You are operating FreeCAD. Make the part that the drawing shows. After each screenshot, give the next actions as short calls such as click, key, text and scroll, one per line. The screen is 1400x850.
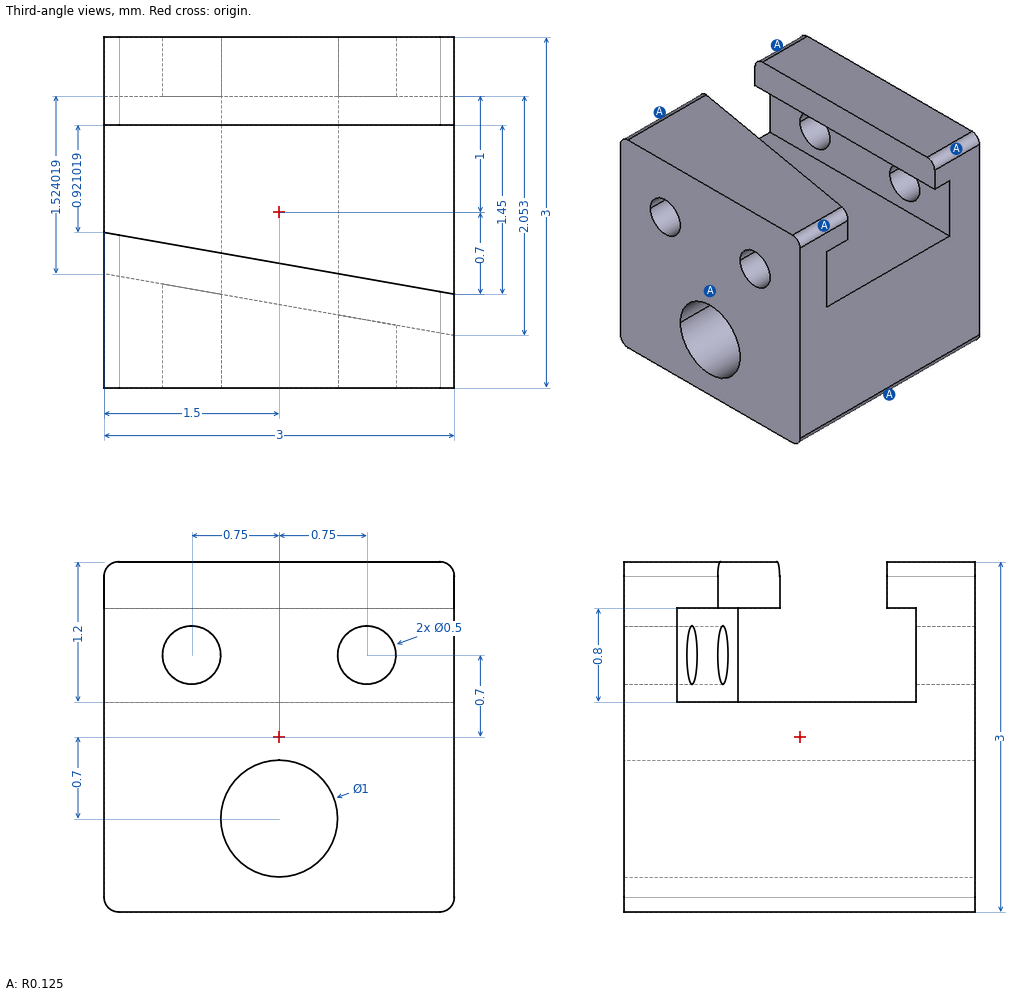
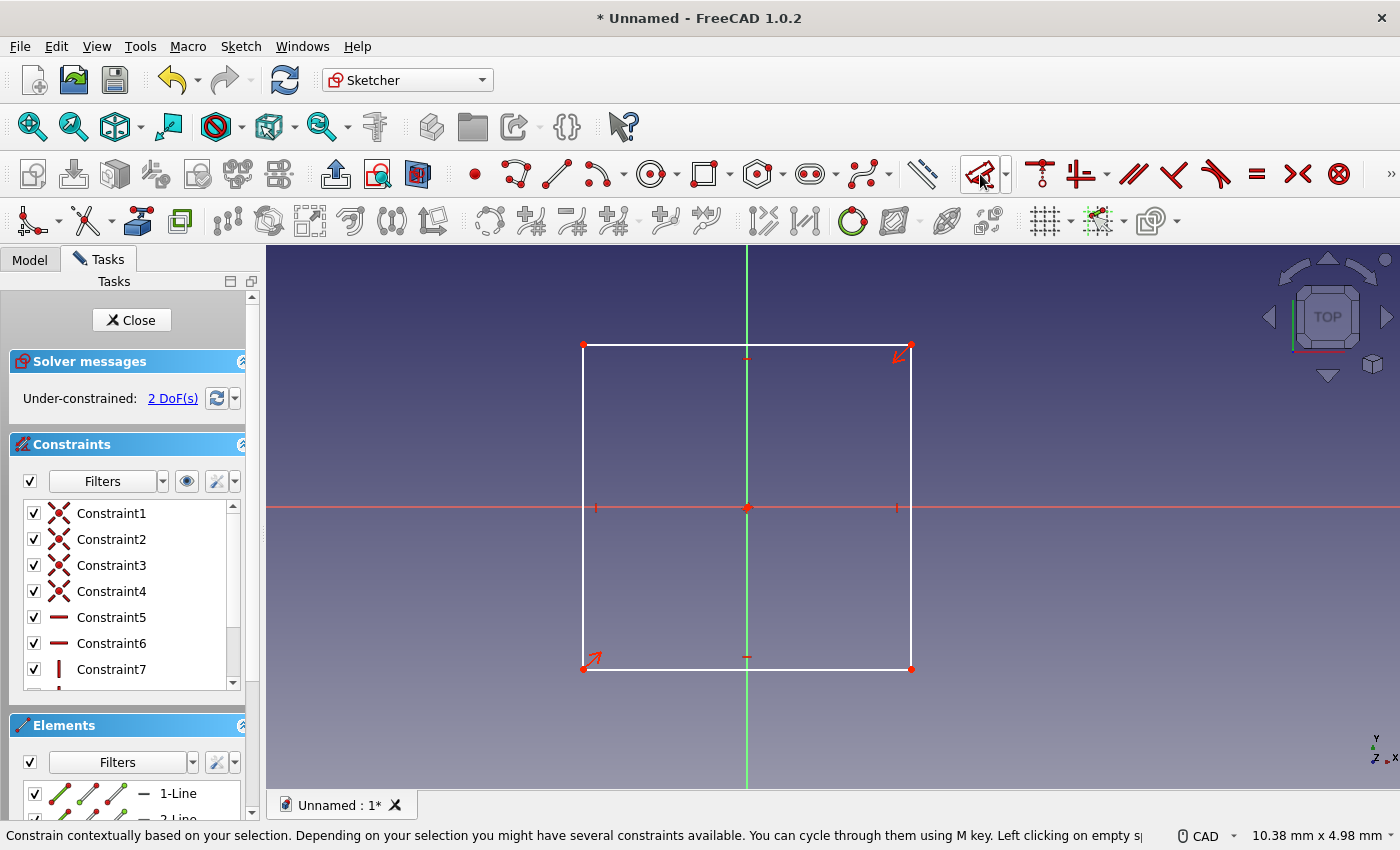
click(681, 670)
click(672, 704)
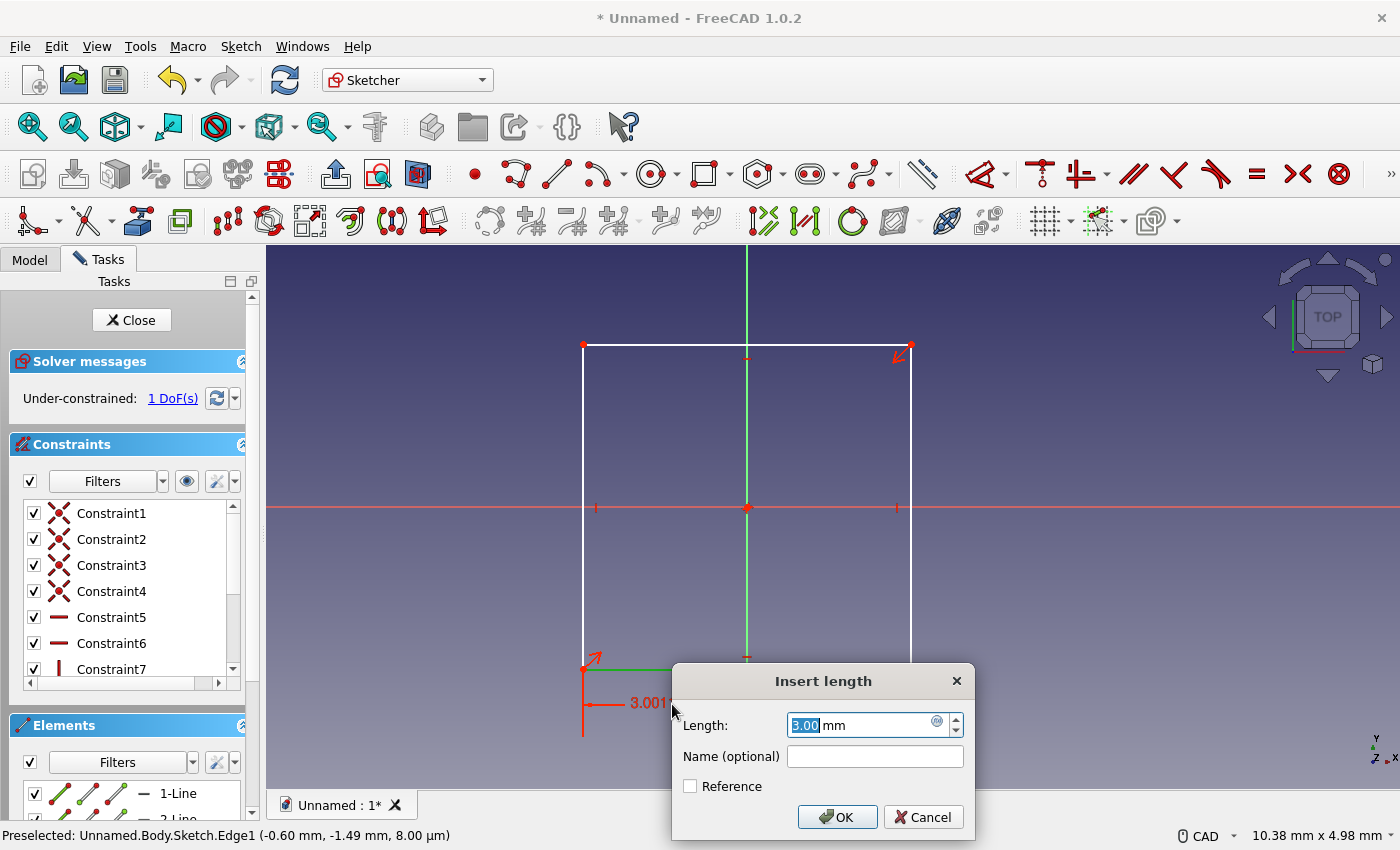
text(3)
key(Return)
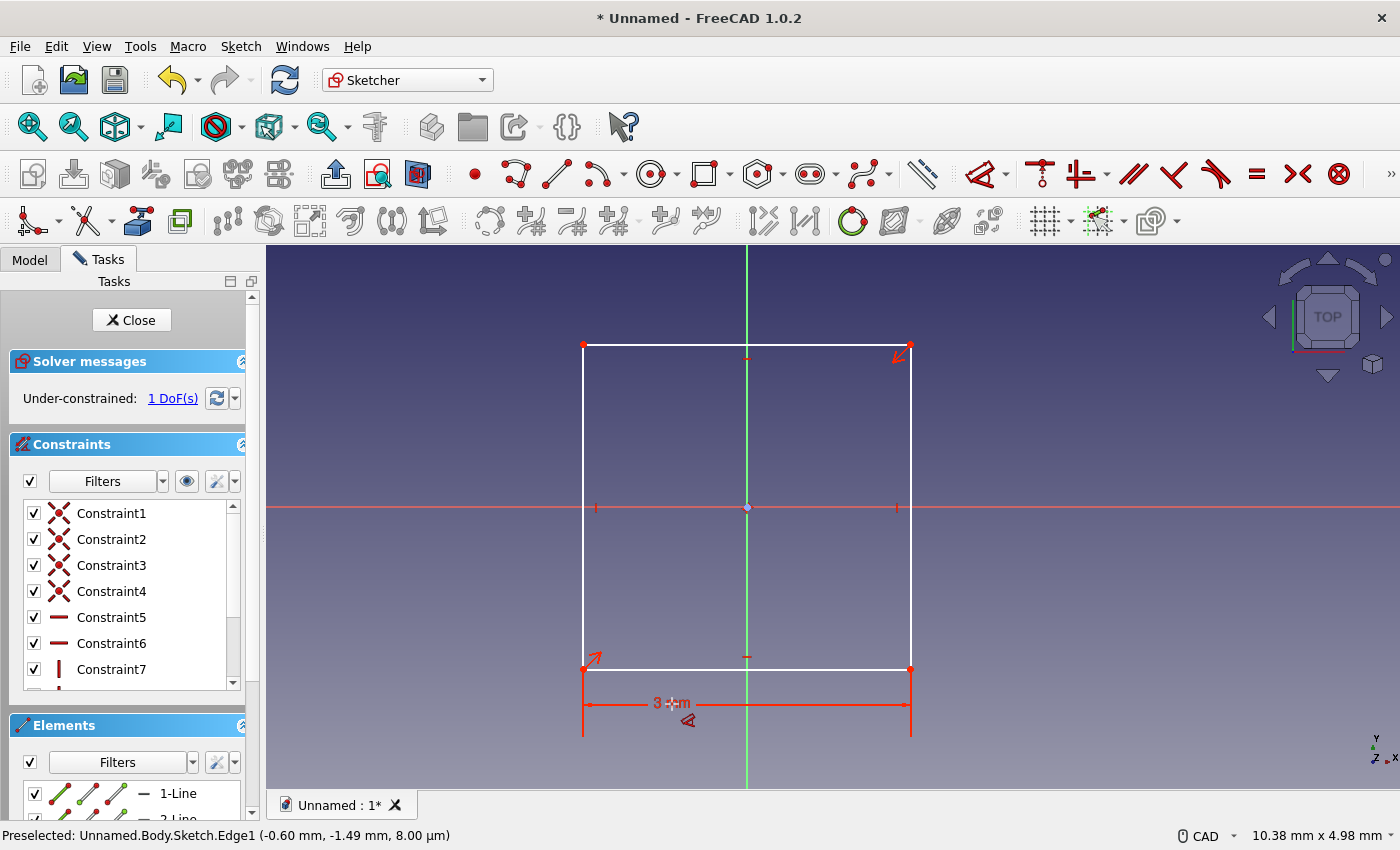
click(911, 572)
click(945, 433)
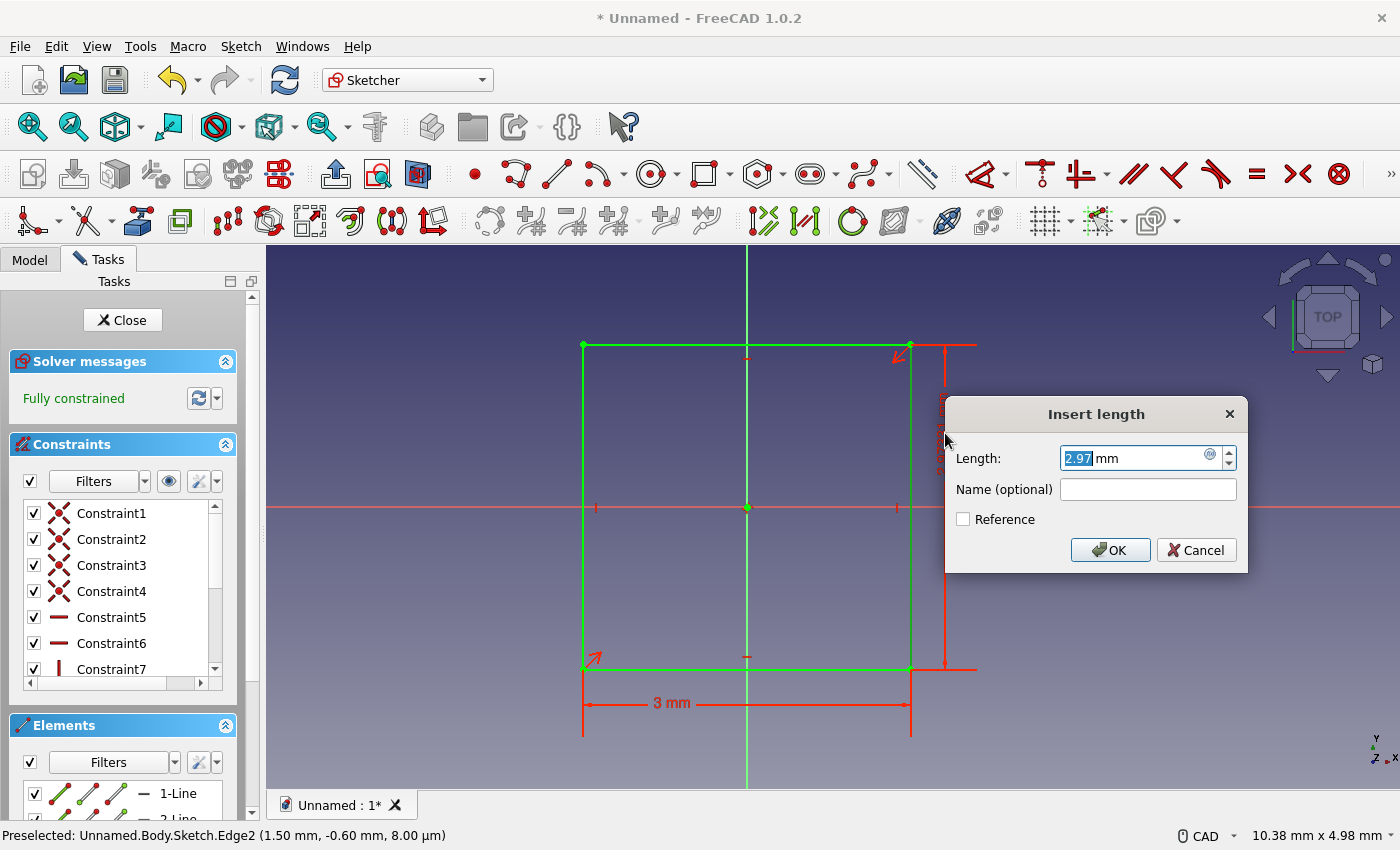
text(3)
key(Return)
key(Escape)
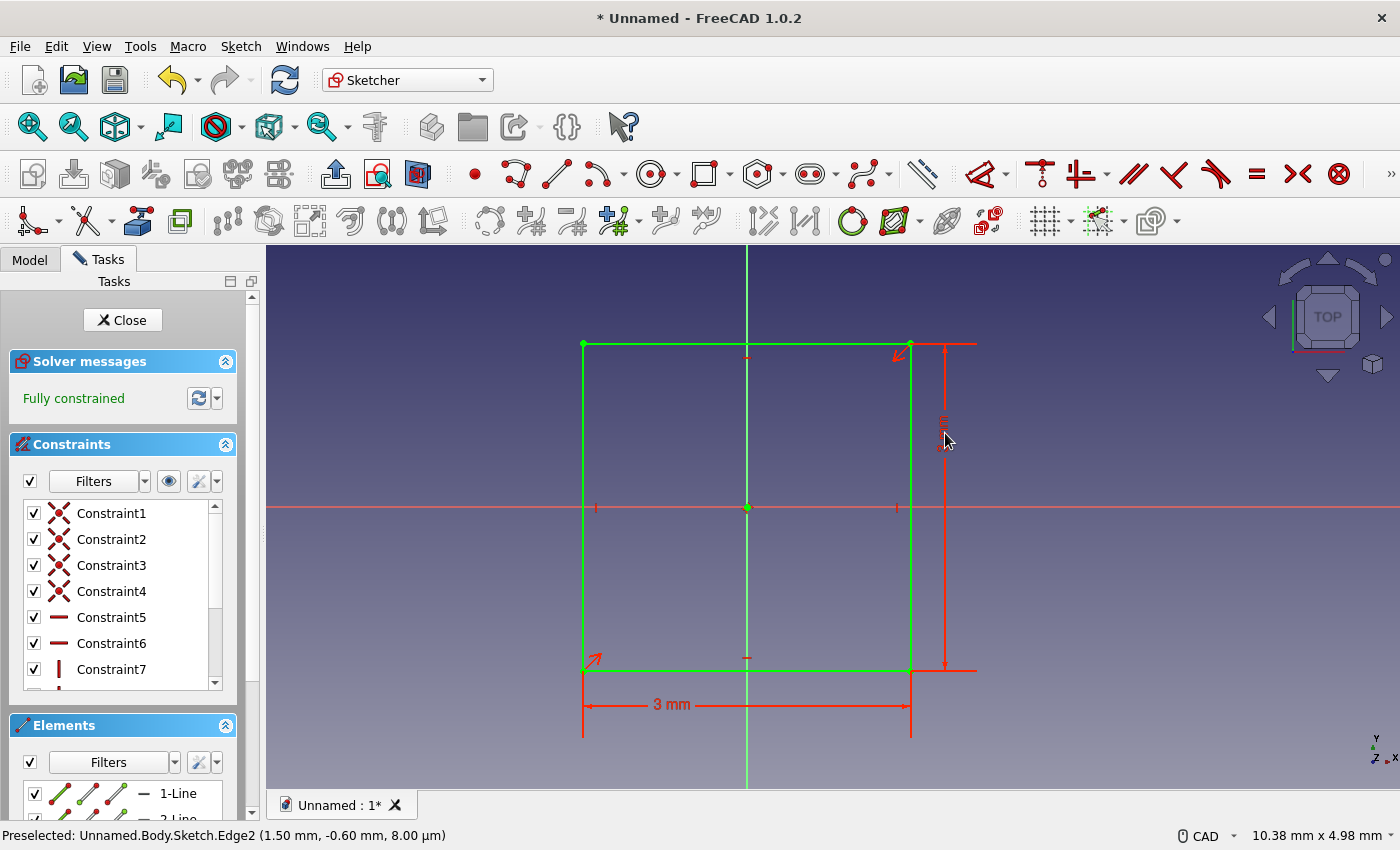
click(123, 320)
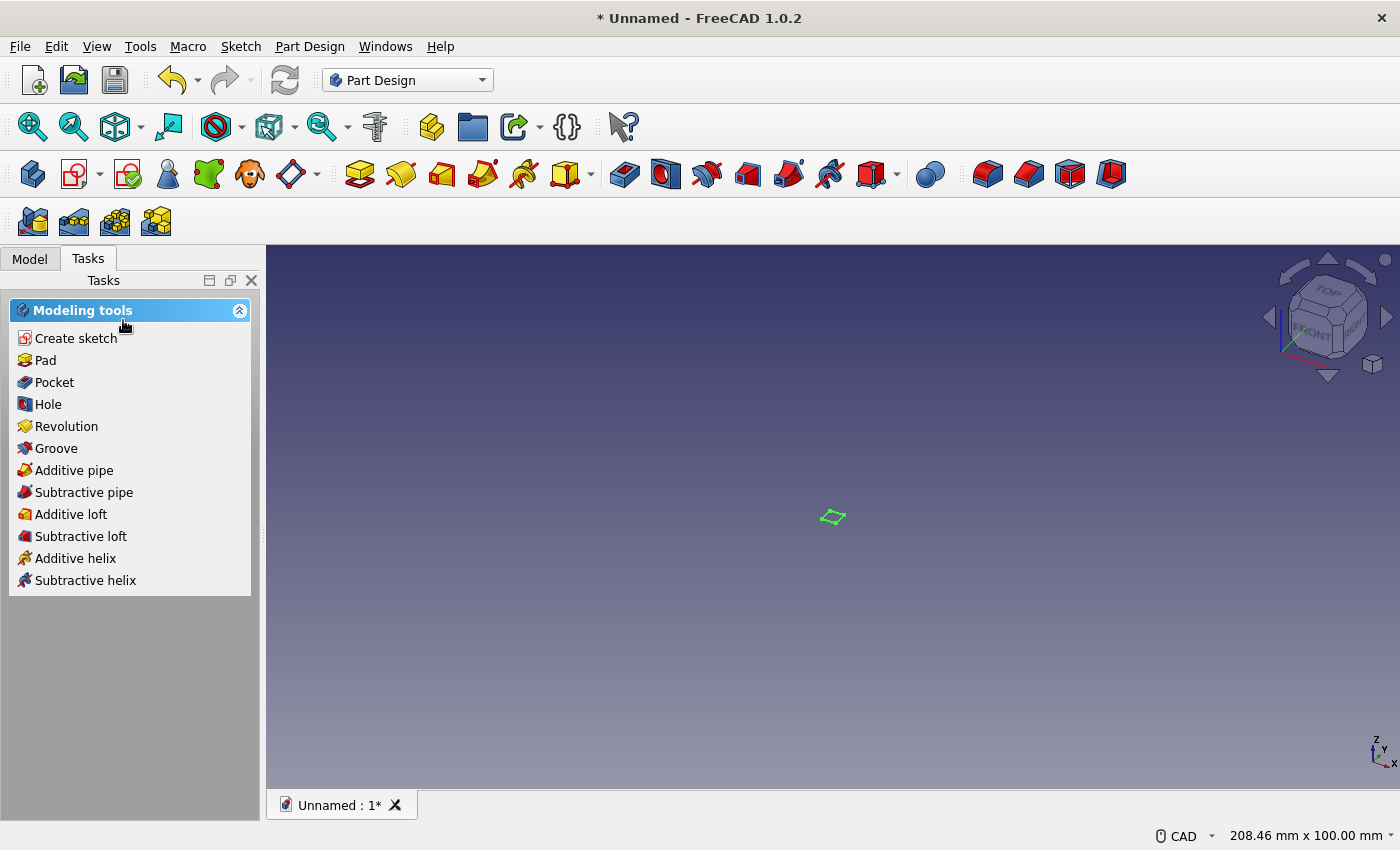
click(360, 174)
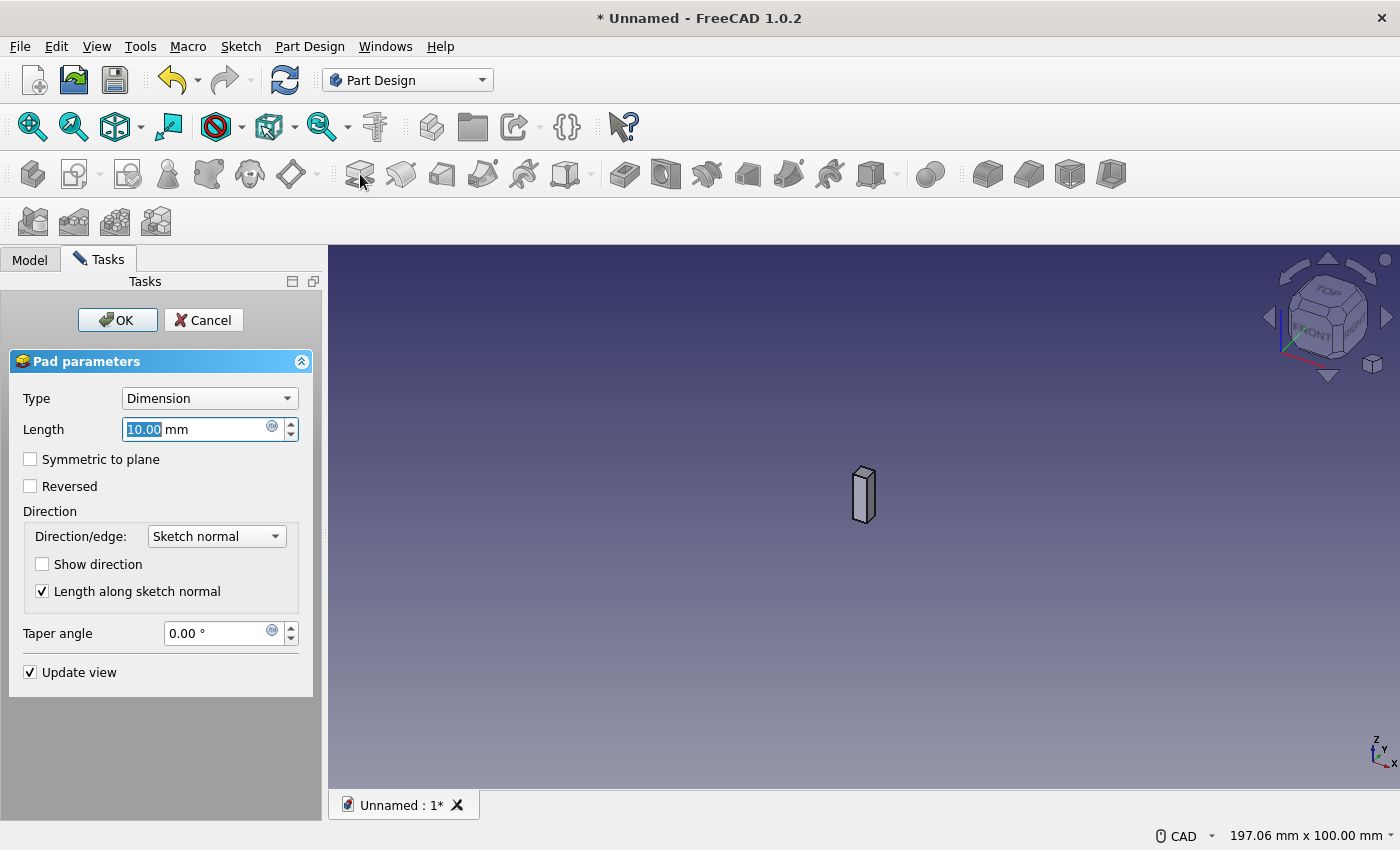
text(3)
key(Tab)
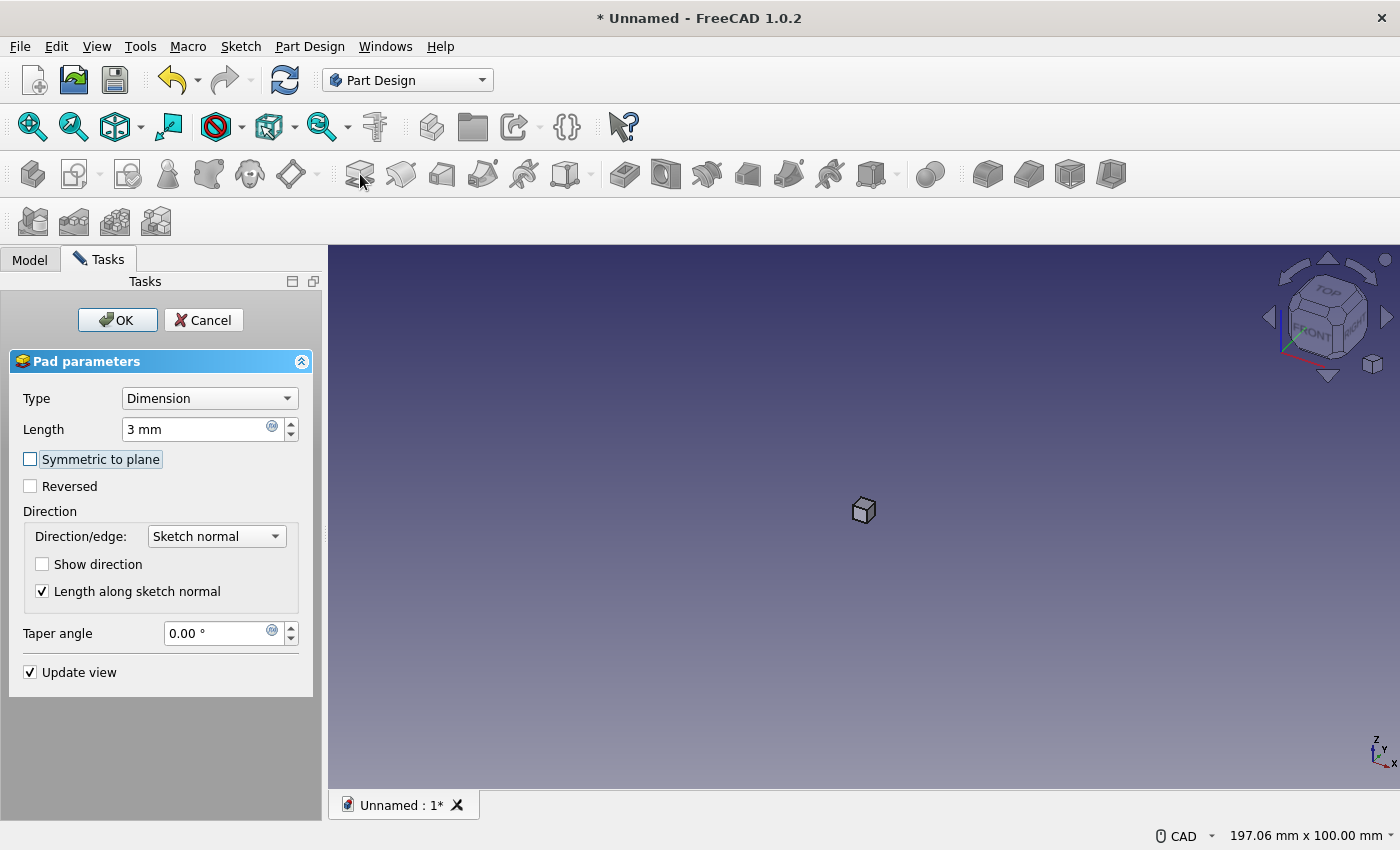
click(31, 459)